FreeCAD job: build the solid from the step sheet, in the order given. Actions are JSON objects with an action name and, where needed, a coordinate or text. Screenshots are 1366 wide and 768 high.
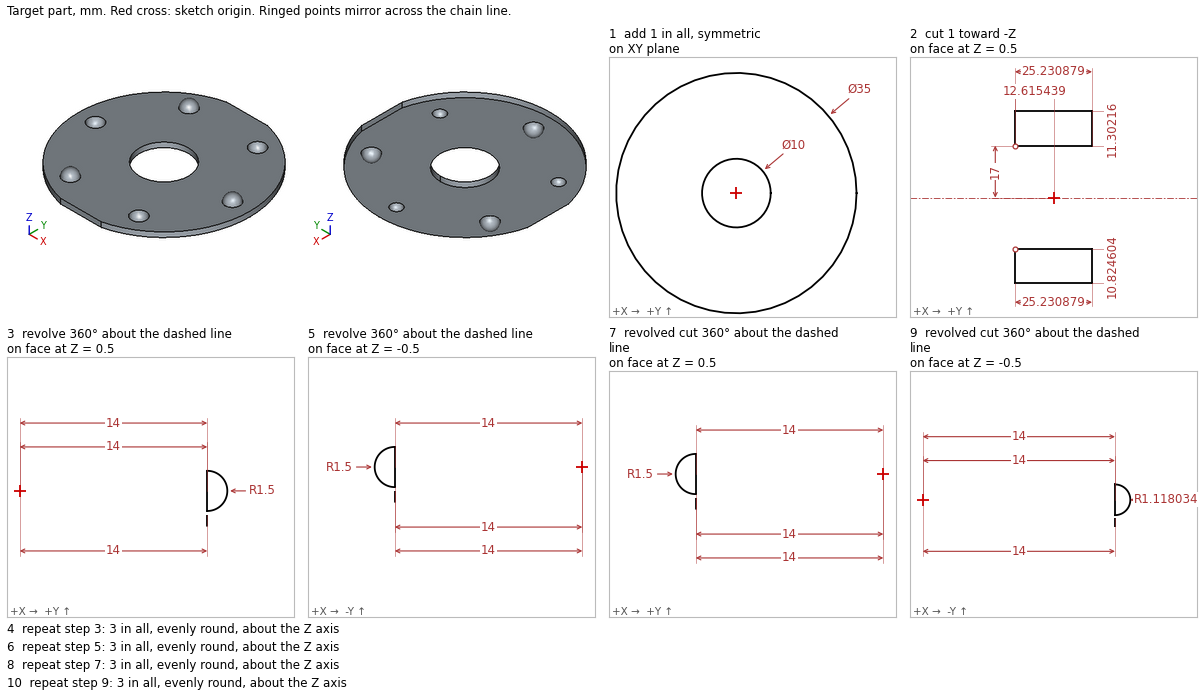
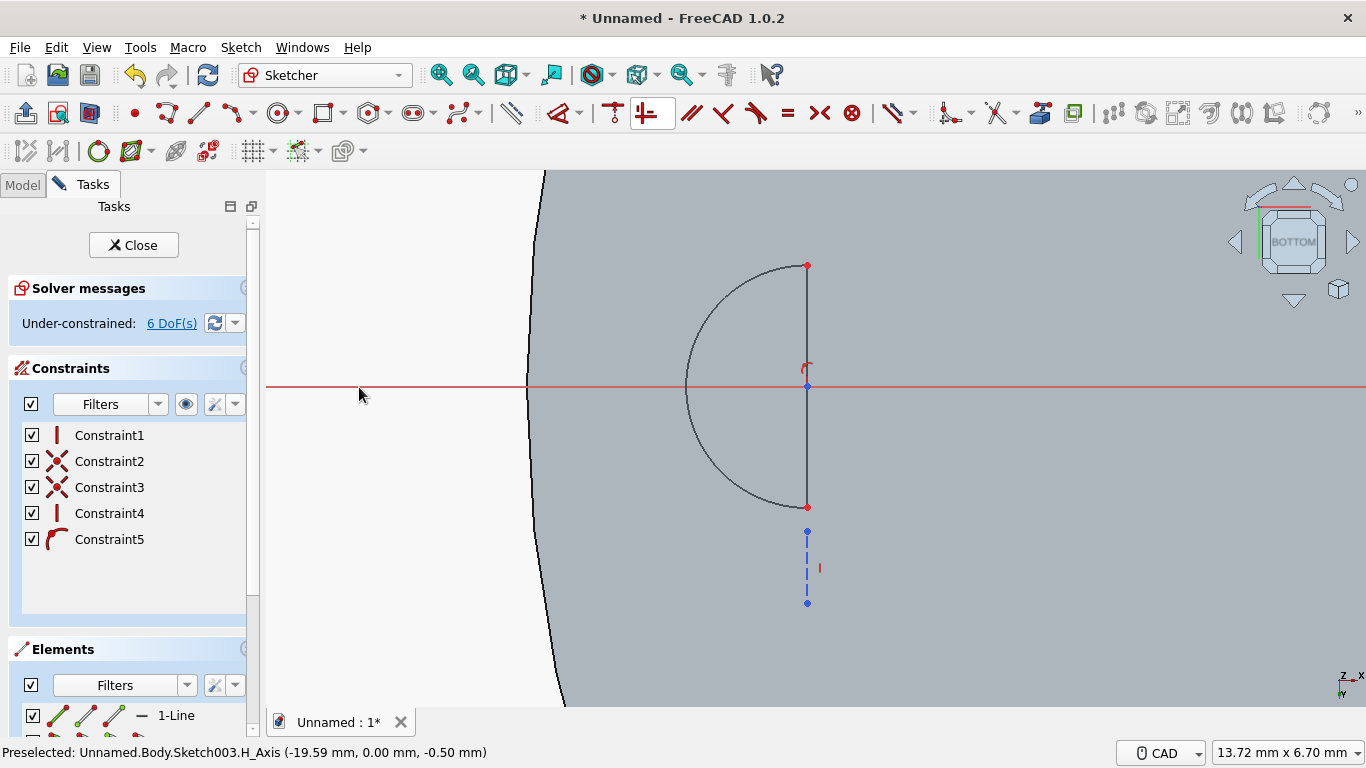
{"action": "key", "text": "d"}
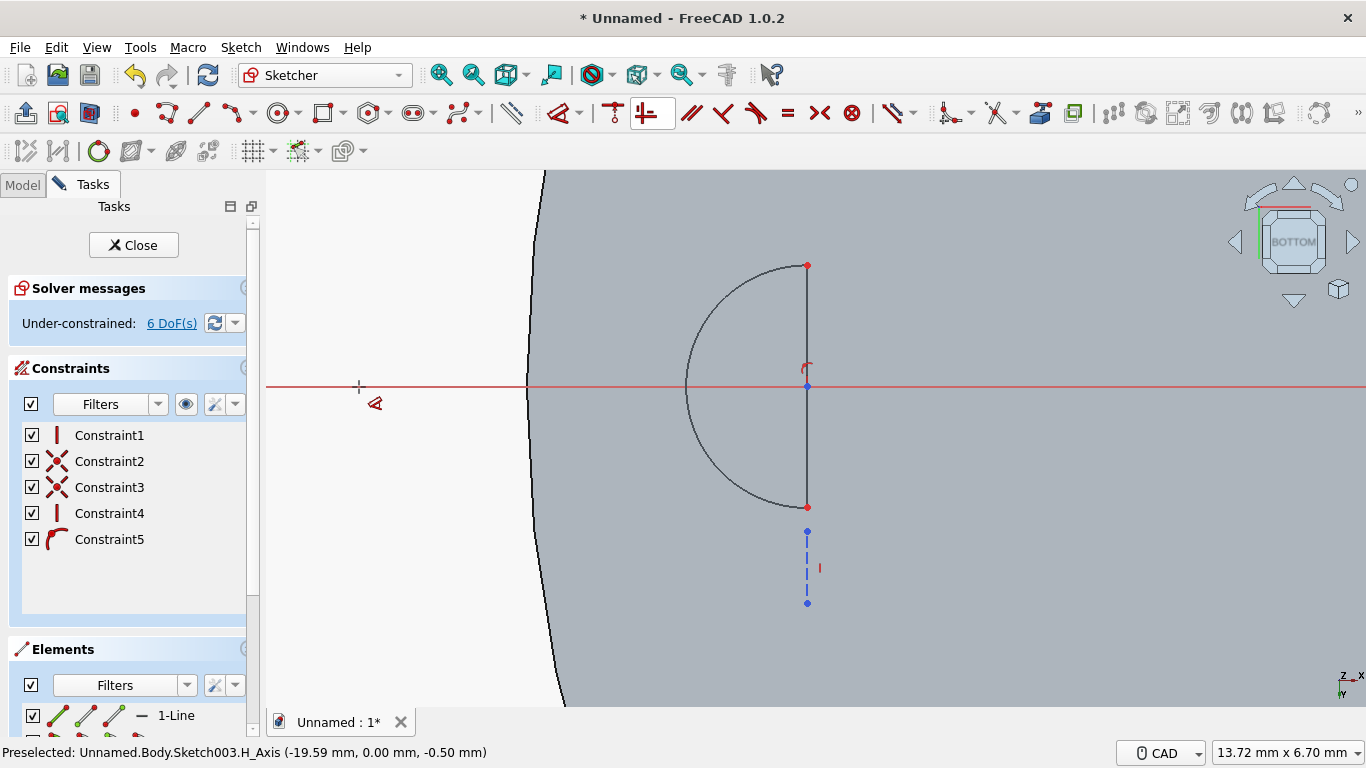
{"action": "left_click", "coordinate": [709, 316]}
{"action": "left_click", "coordinate": [683, 297]}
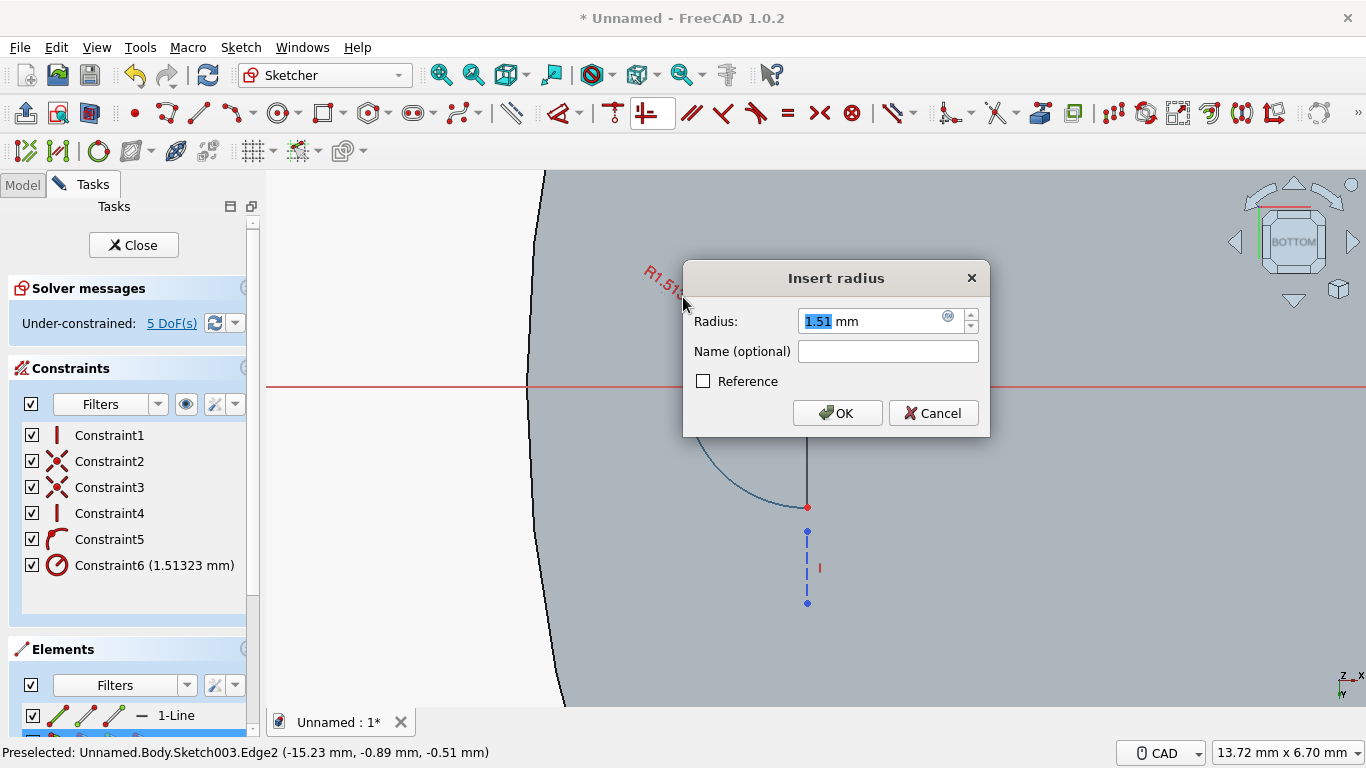
{"action": "type", "text": "1.5"}
{"action": "key", "text": "Return"}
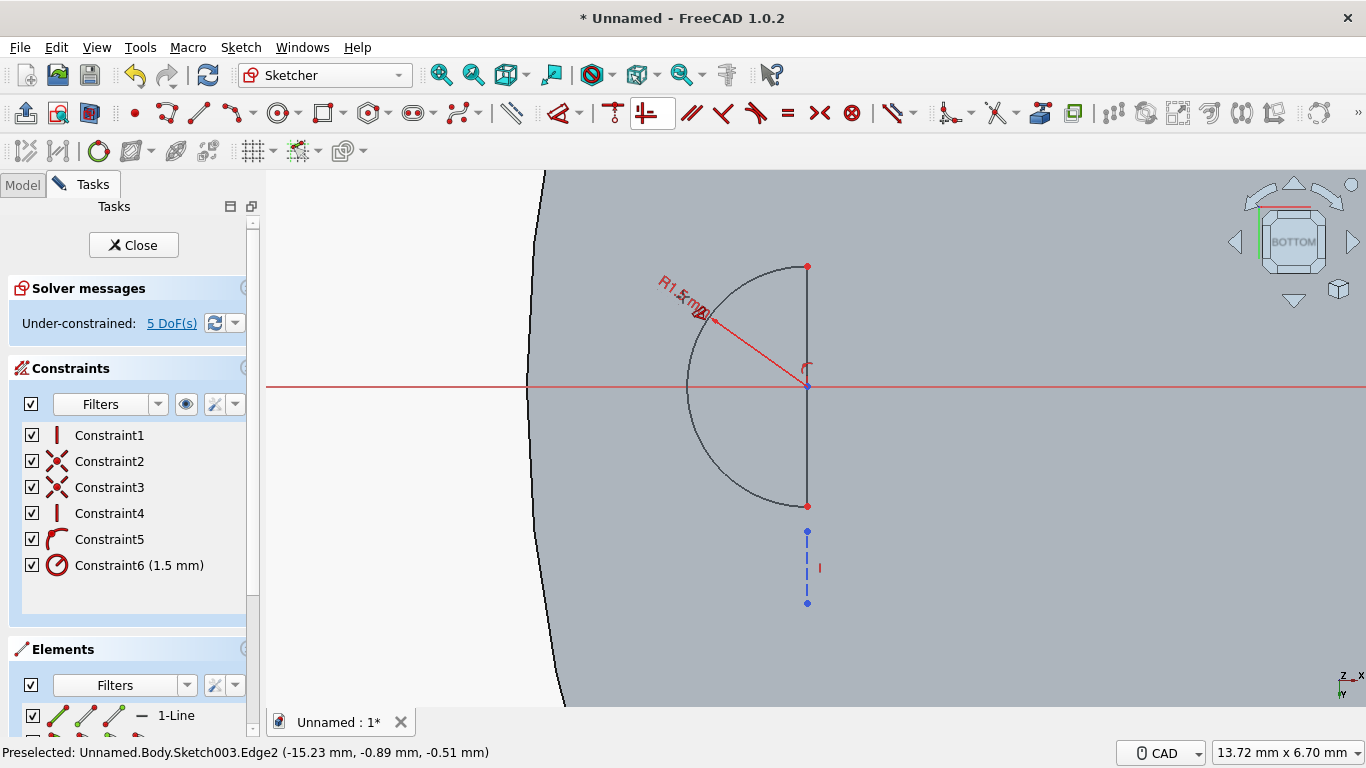
{"action": "left_click", "coordinate": [807, 507]}
{"action": "left_click", "coordinate": [1004, 541]}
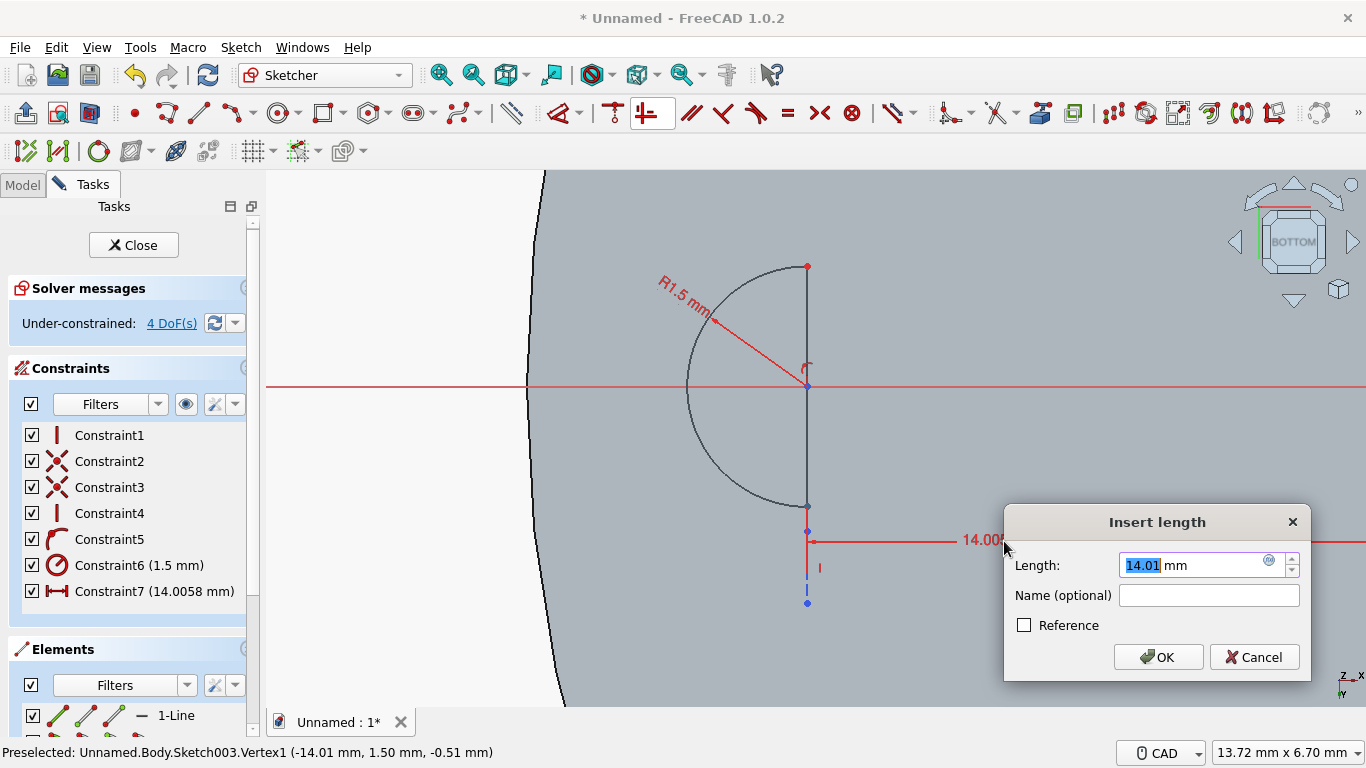
{"action": "type", "text": "14"}
{"action": "key", "text": "Return"}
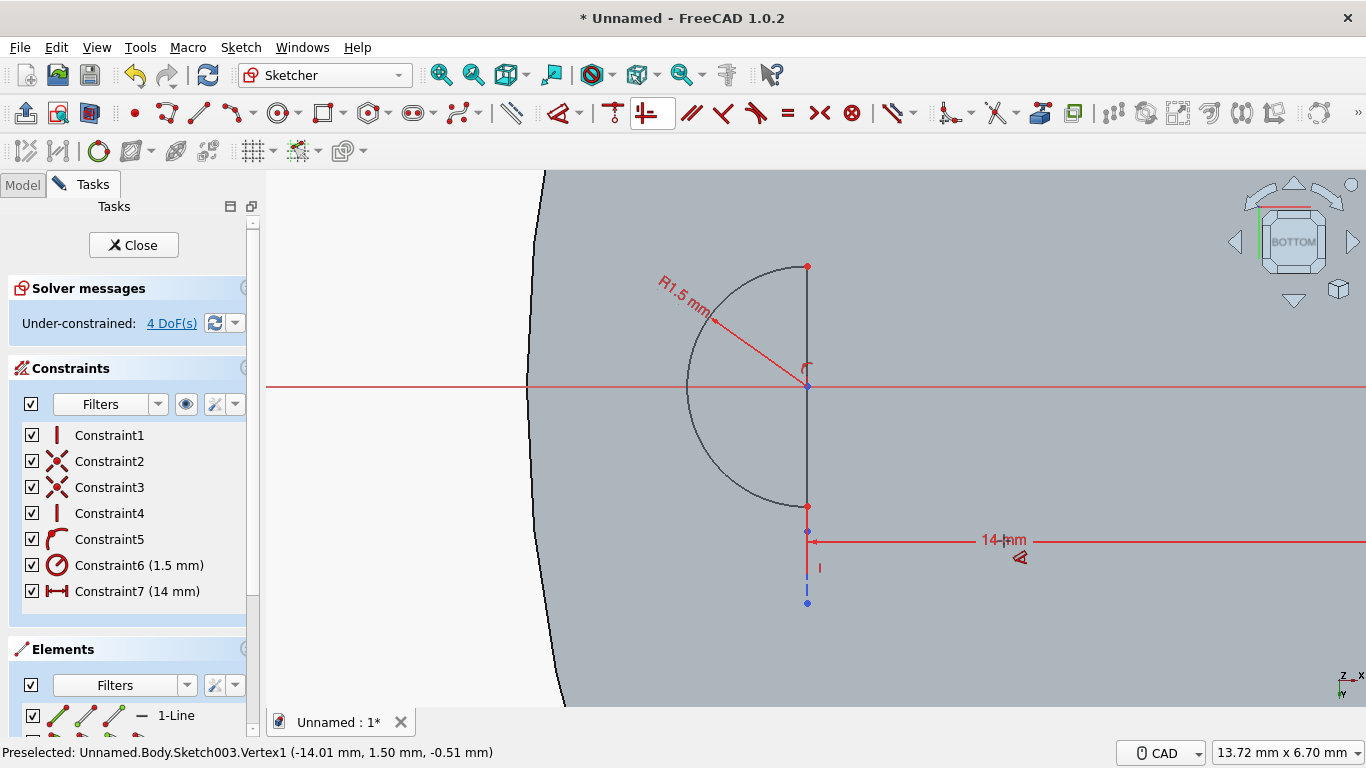
{"action": "left_click", "coordinate": [807, 532]}
{"action": "left_click", "coordinate": [1004, 566]}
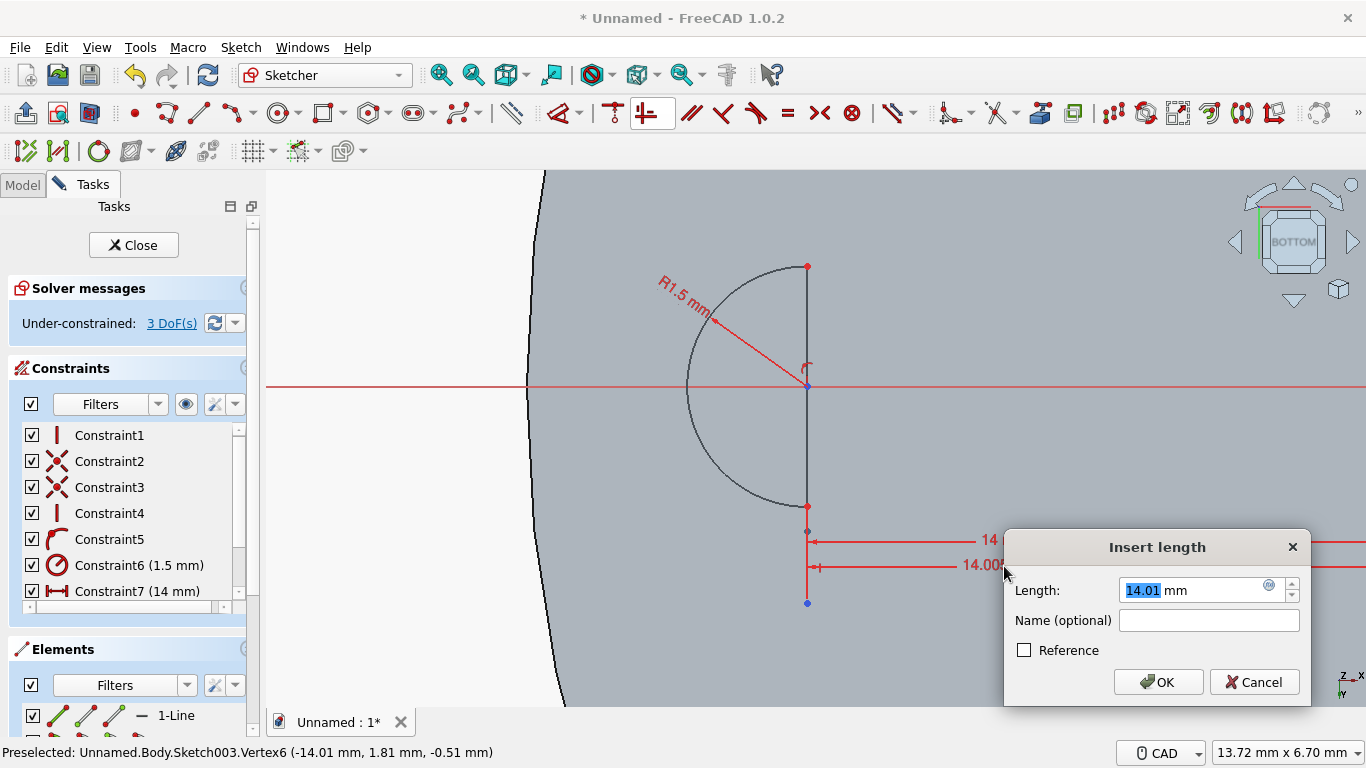
{"action": "type", "text": "14"}
{"action": "key", "text": "Return"}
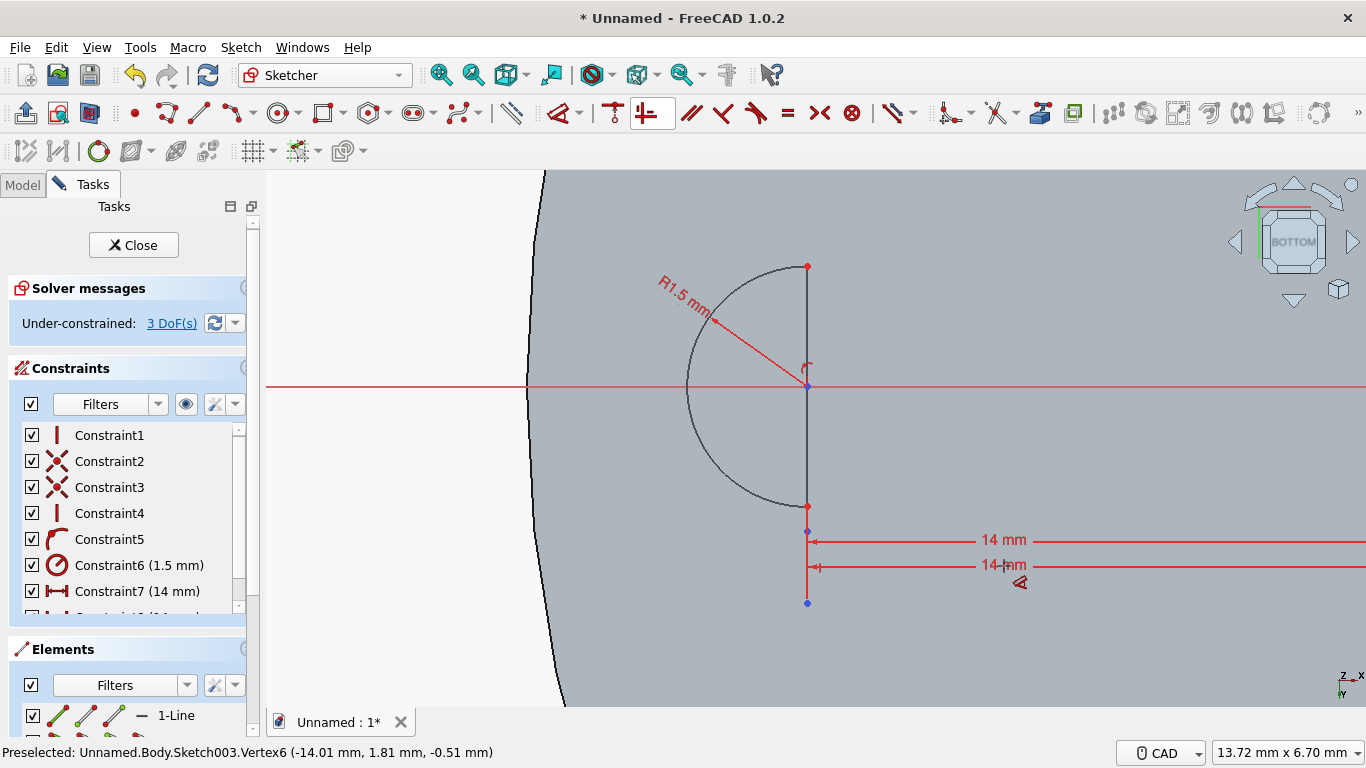
{"action": "left_click", "coordinate": [808, 387]}
{"action": "left_click", "coordinate": [1004, 353]}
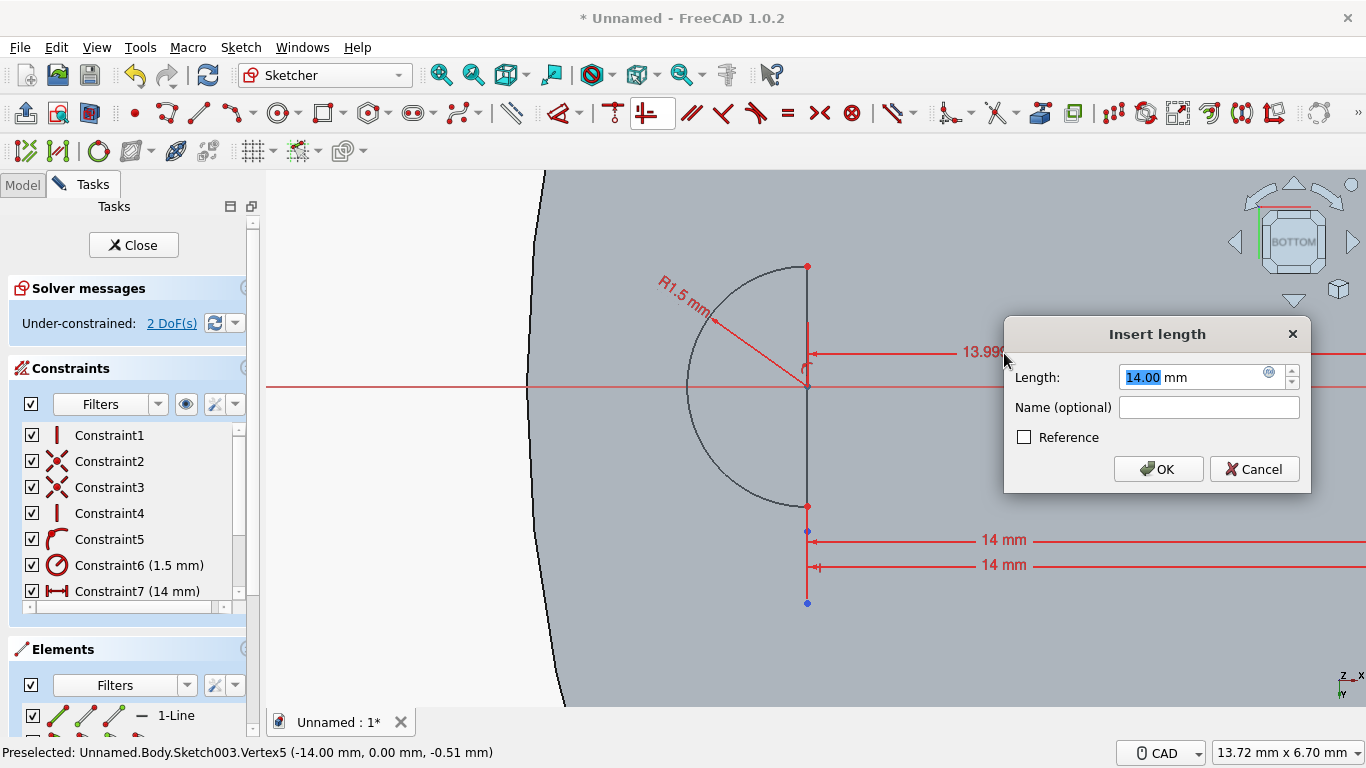
{"action": "type", "text": "14"}
{"action": "key", "text": "Return"}
{"action": "key", "text": "Escape"}